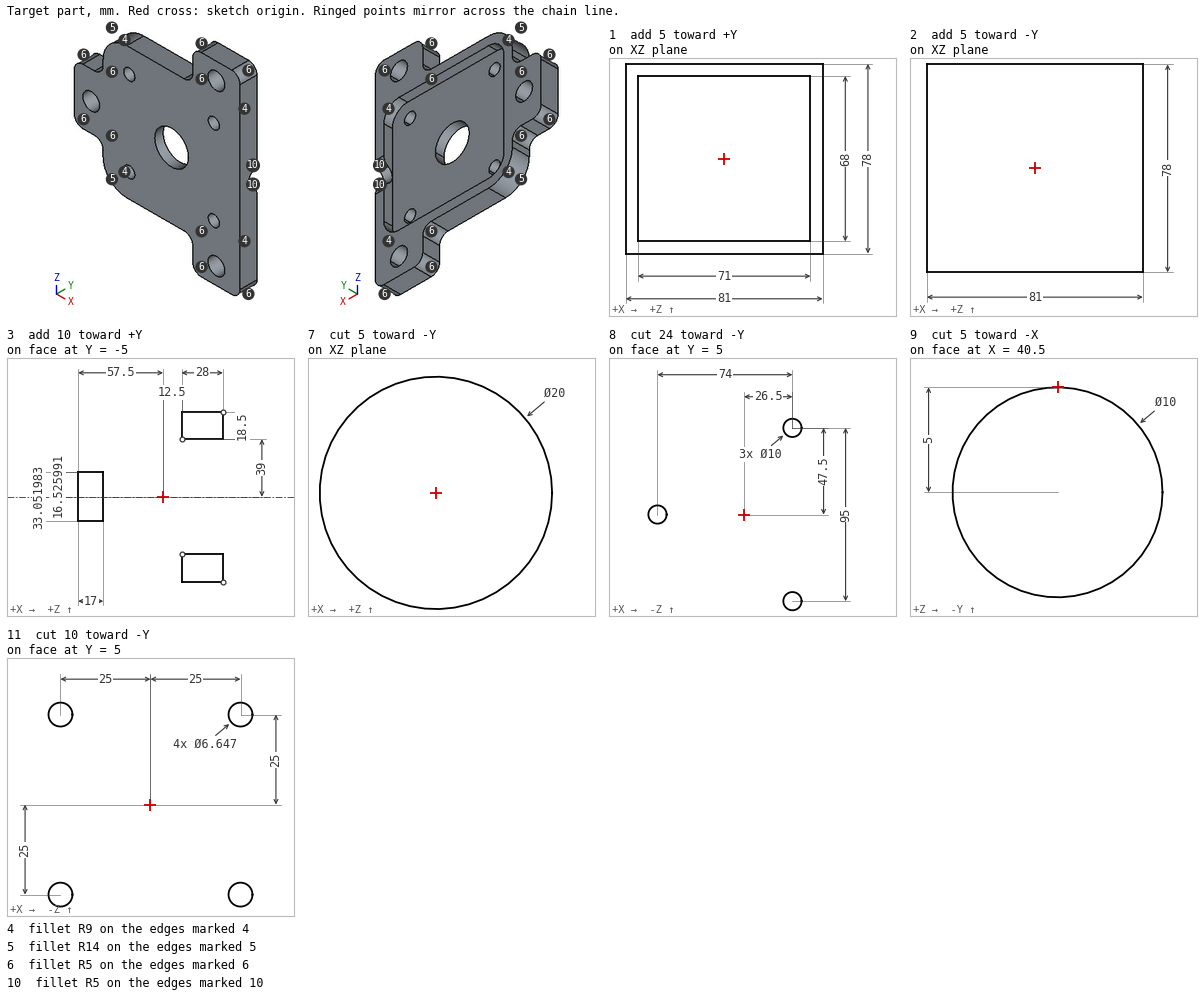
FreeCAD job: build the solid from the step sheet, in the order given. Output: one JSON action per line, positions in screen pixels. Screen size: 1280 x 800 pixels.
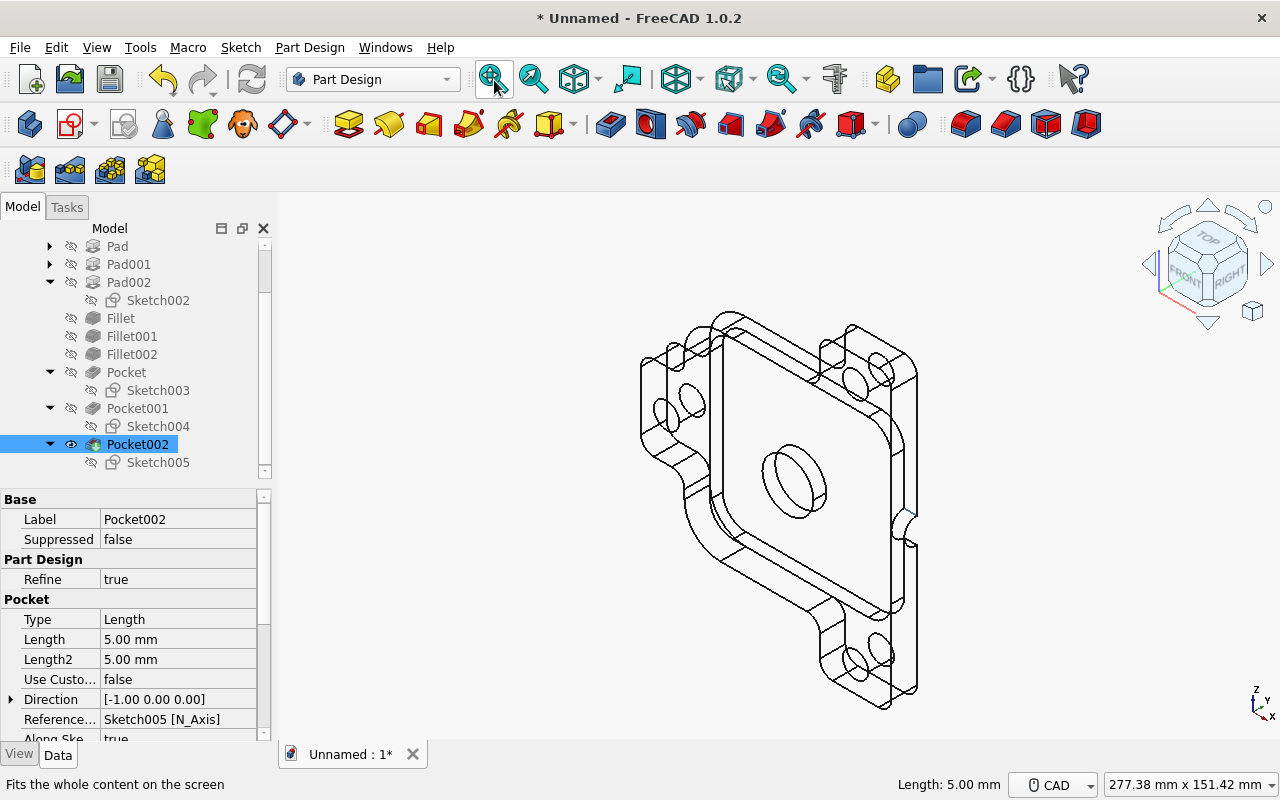
{"action": "scroll", "coordinate": [911, 540], "scroll_direction": "up", "scroll_amount": 4}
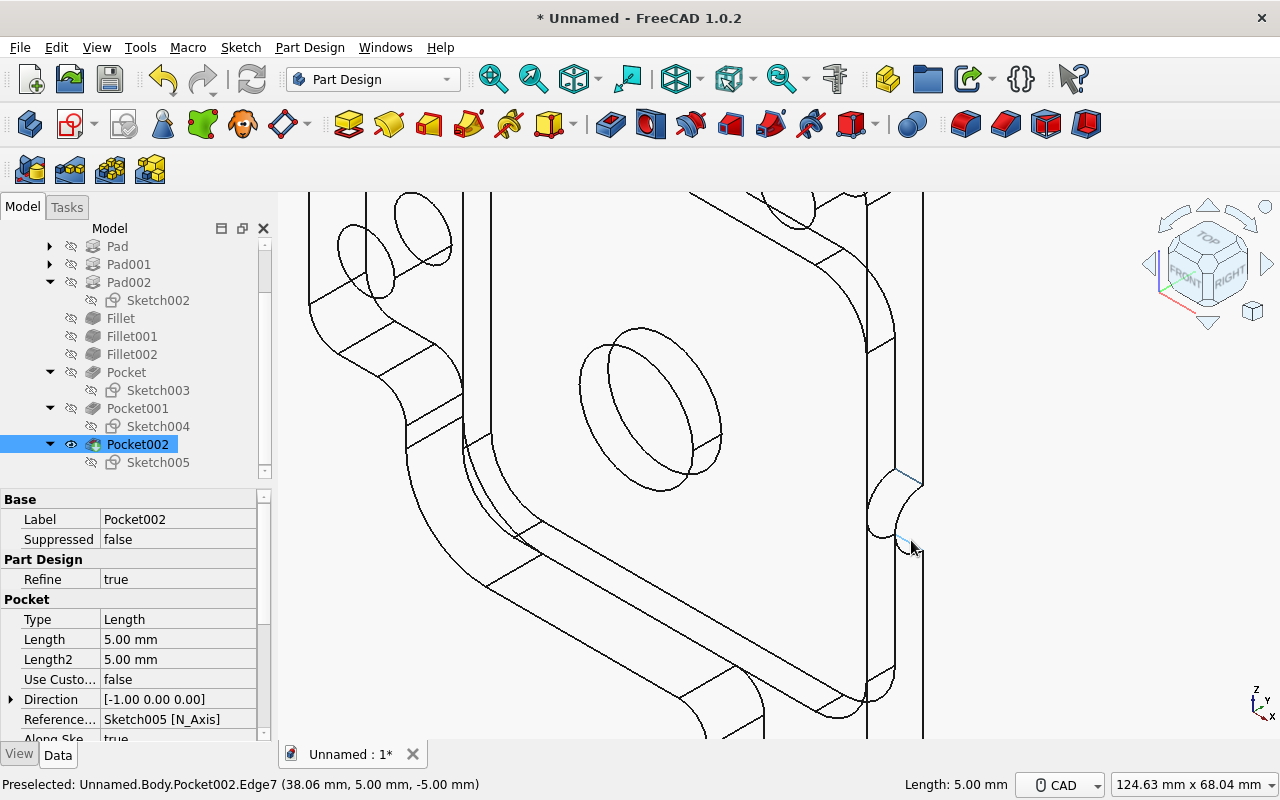
{"action": "left_click", "coordinate": [909, 541], "text": "ctrl"}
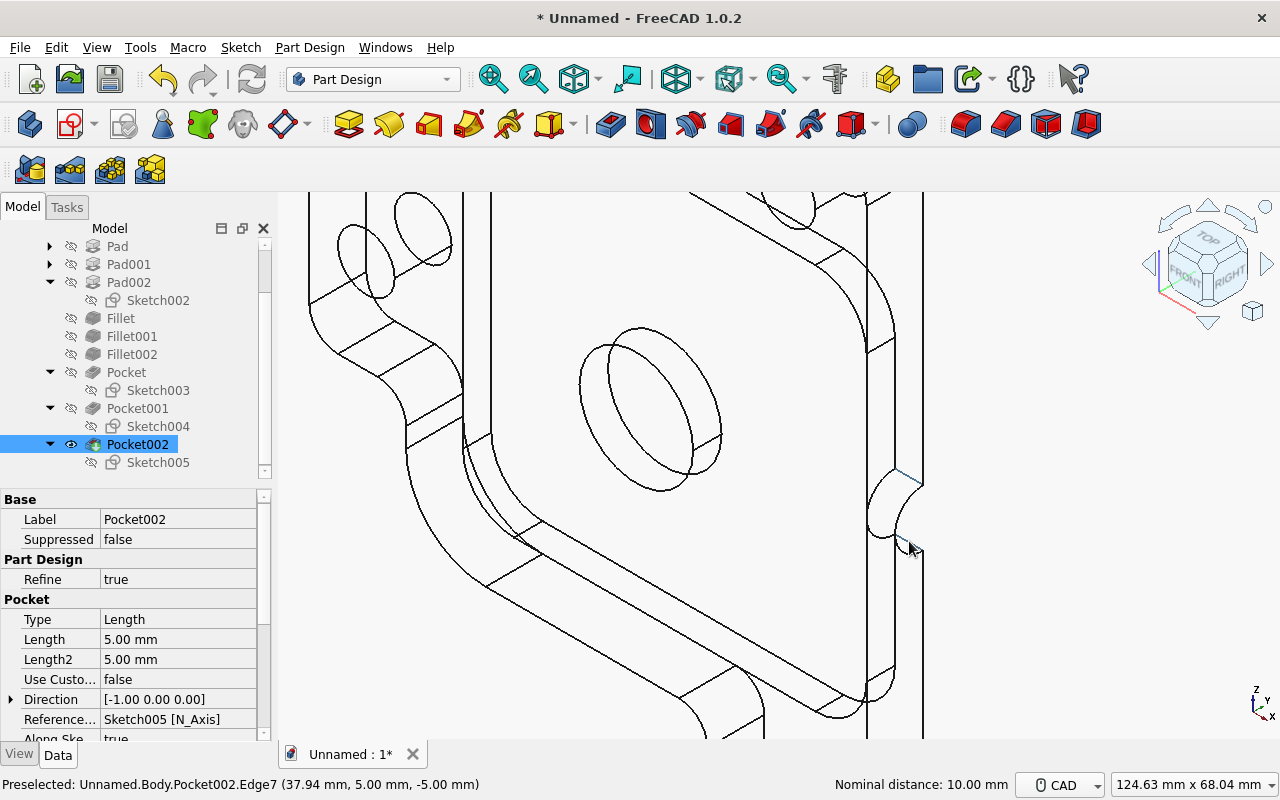
{"action": "key", "text": "v 1"}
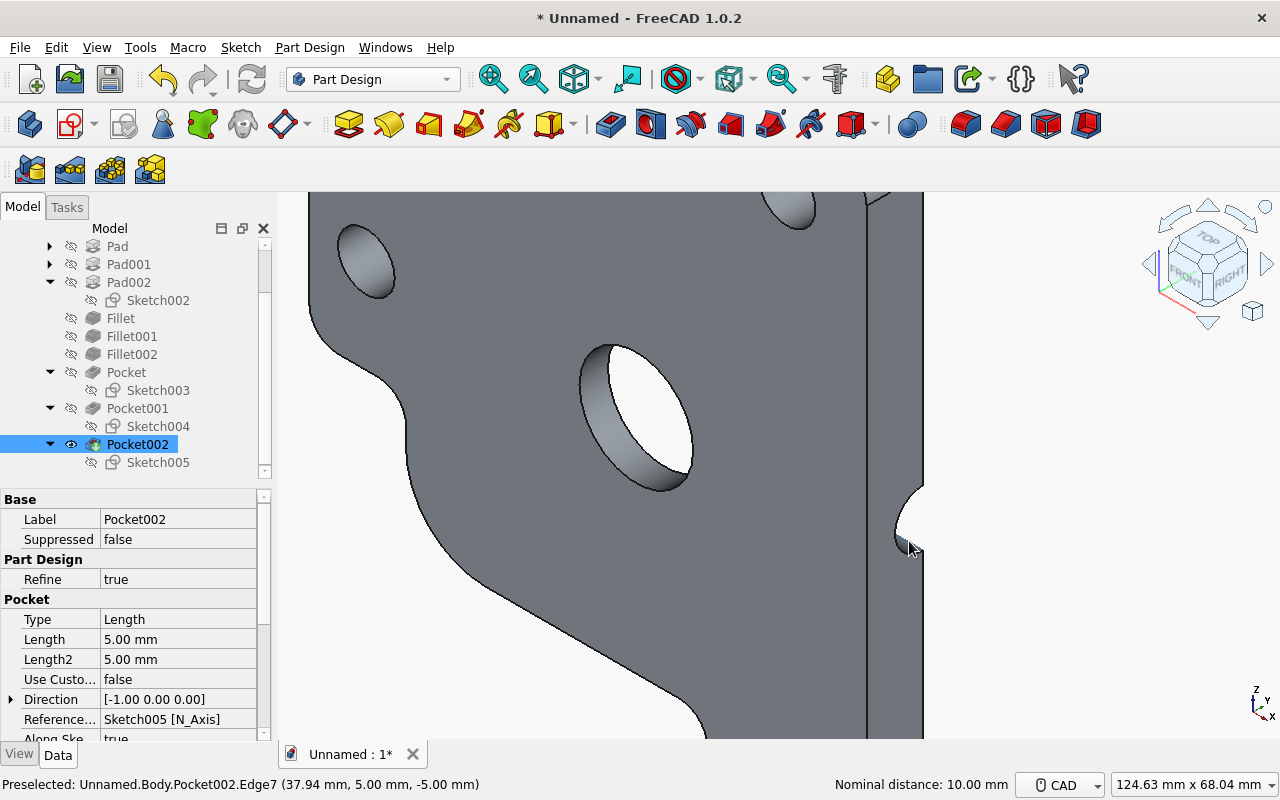
{"action": "left_click", "coordinate": [966, 124]}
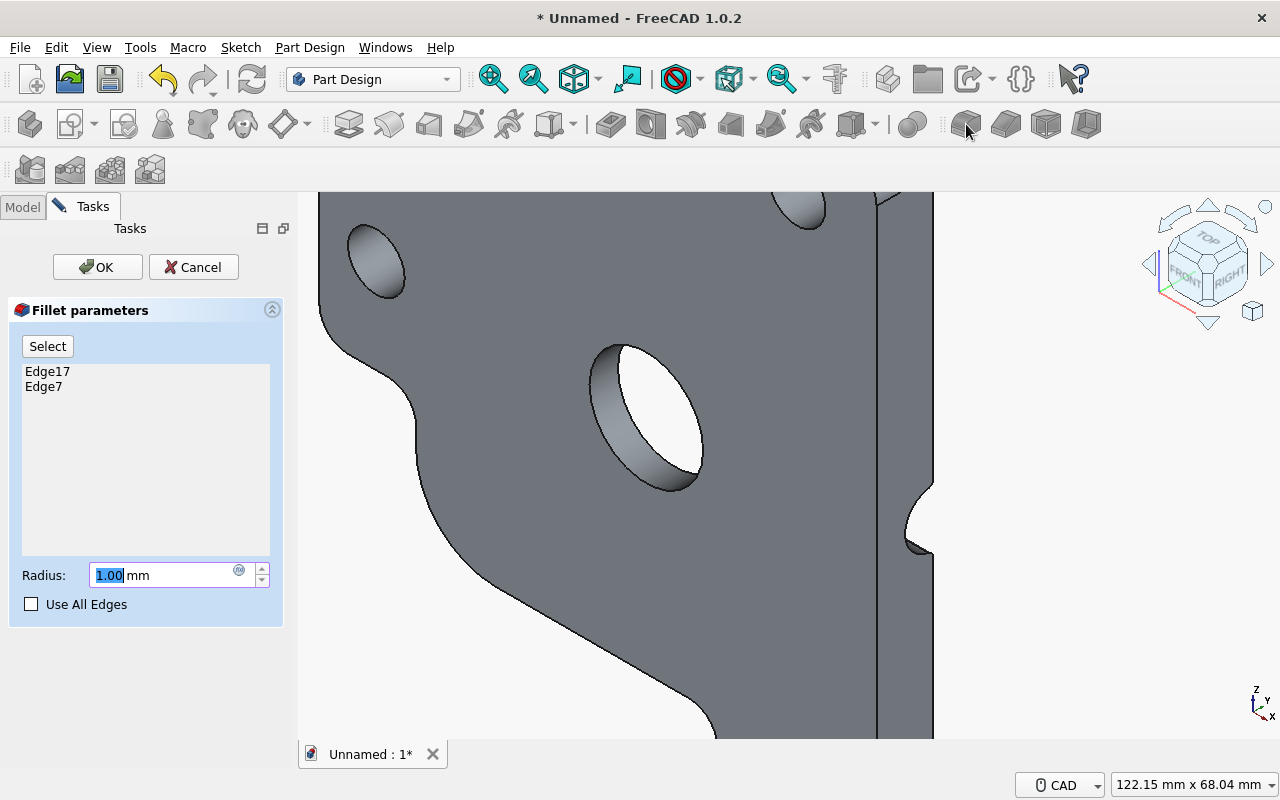
{"action": "type", "text": "5"}
{"action": "key", "text": "Tab"}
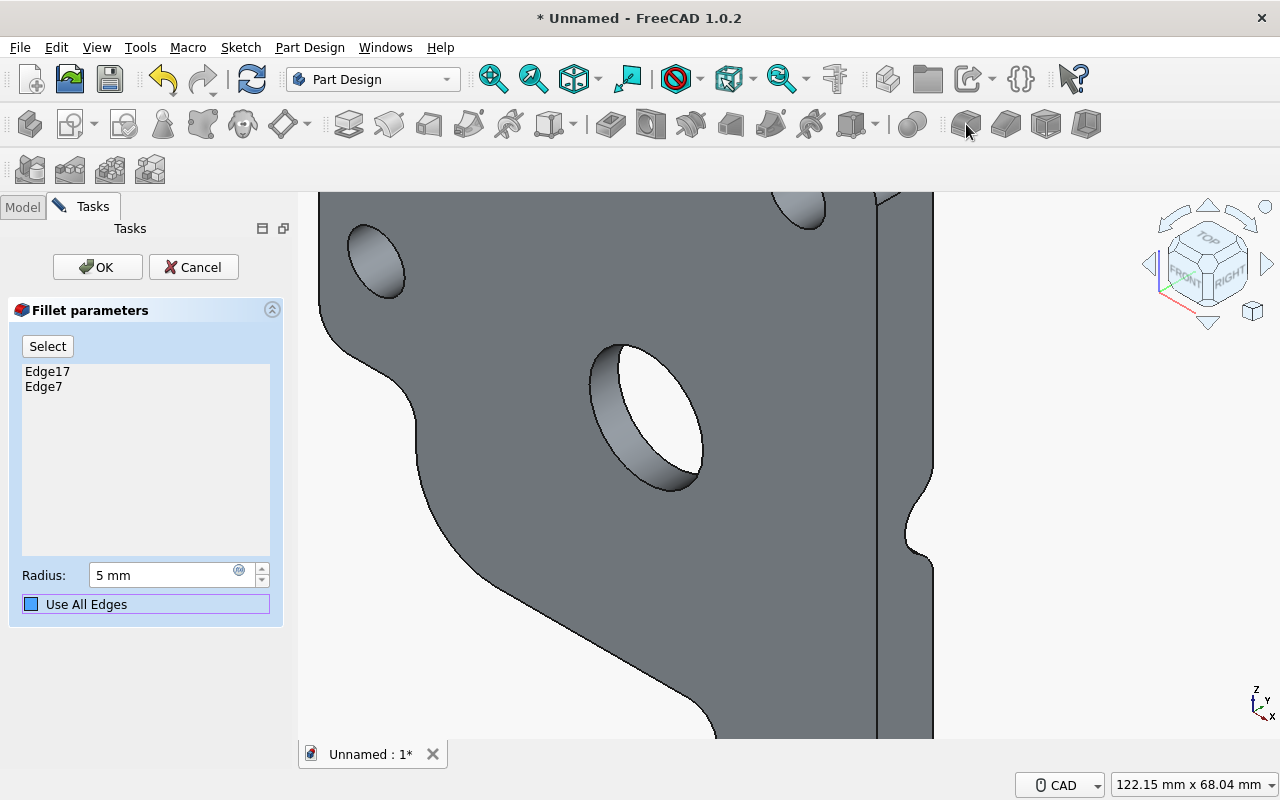
{"action": "left_click", "coordinate": [98, 267]}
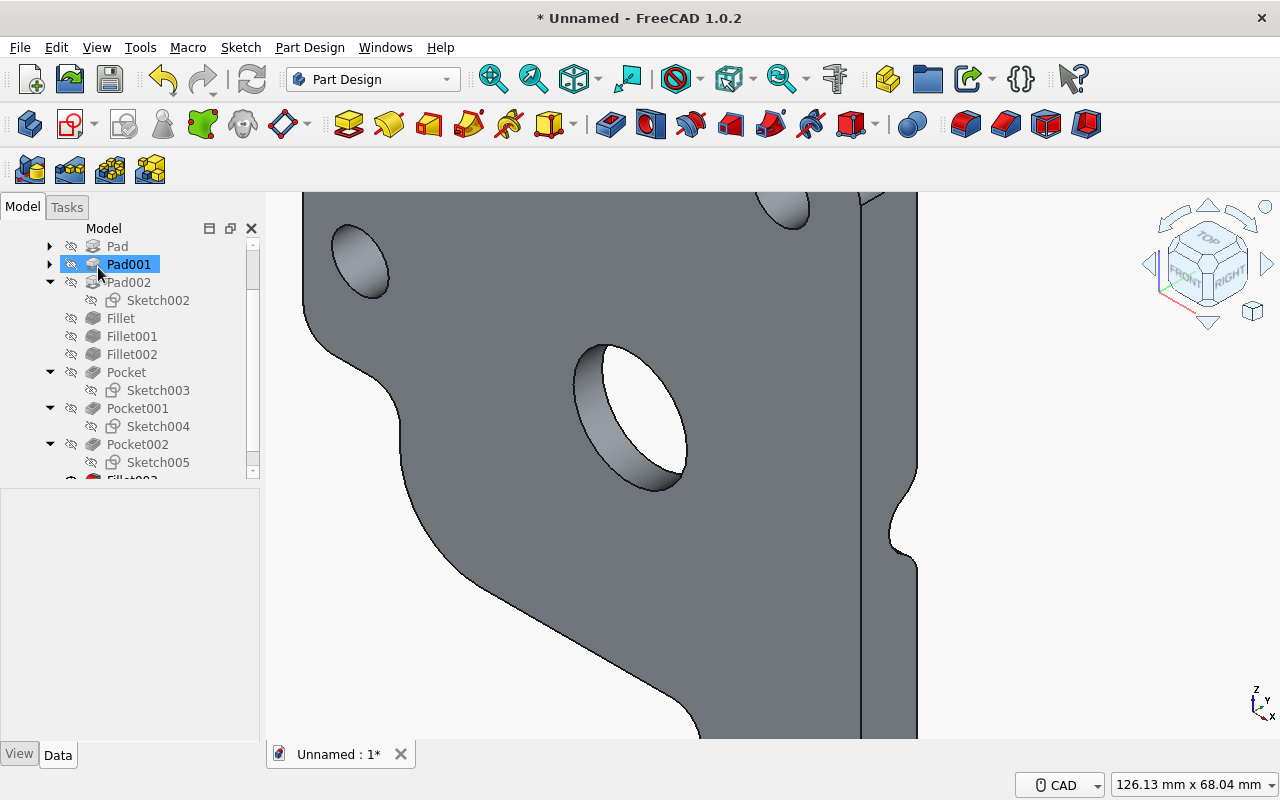
{"action": "key", "text": "v f"}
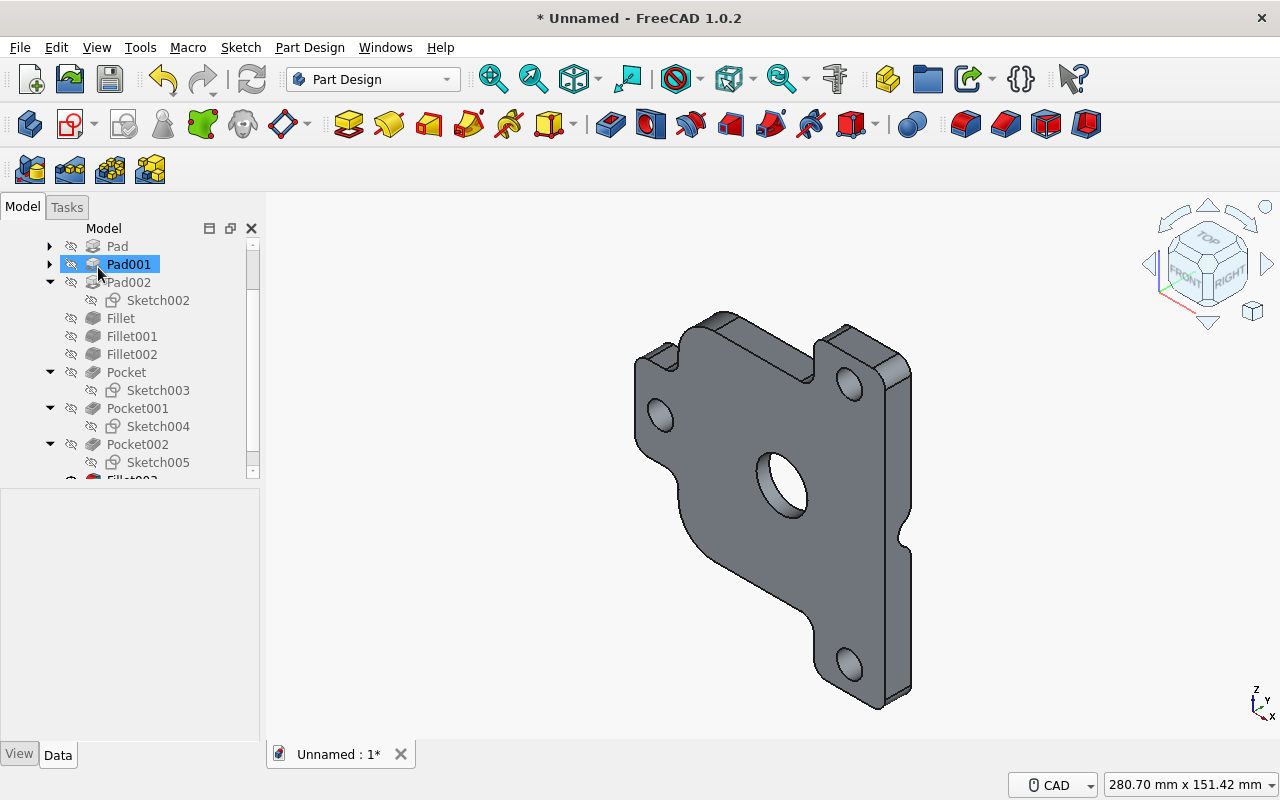
{"action": "key", "text": "4"}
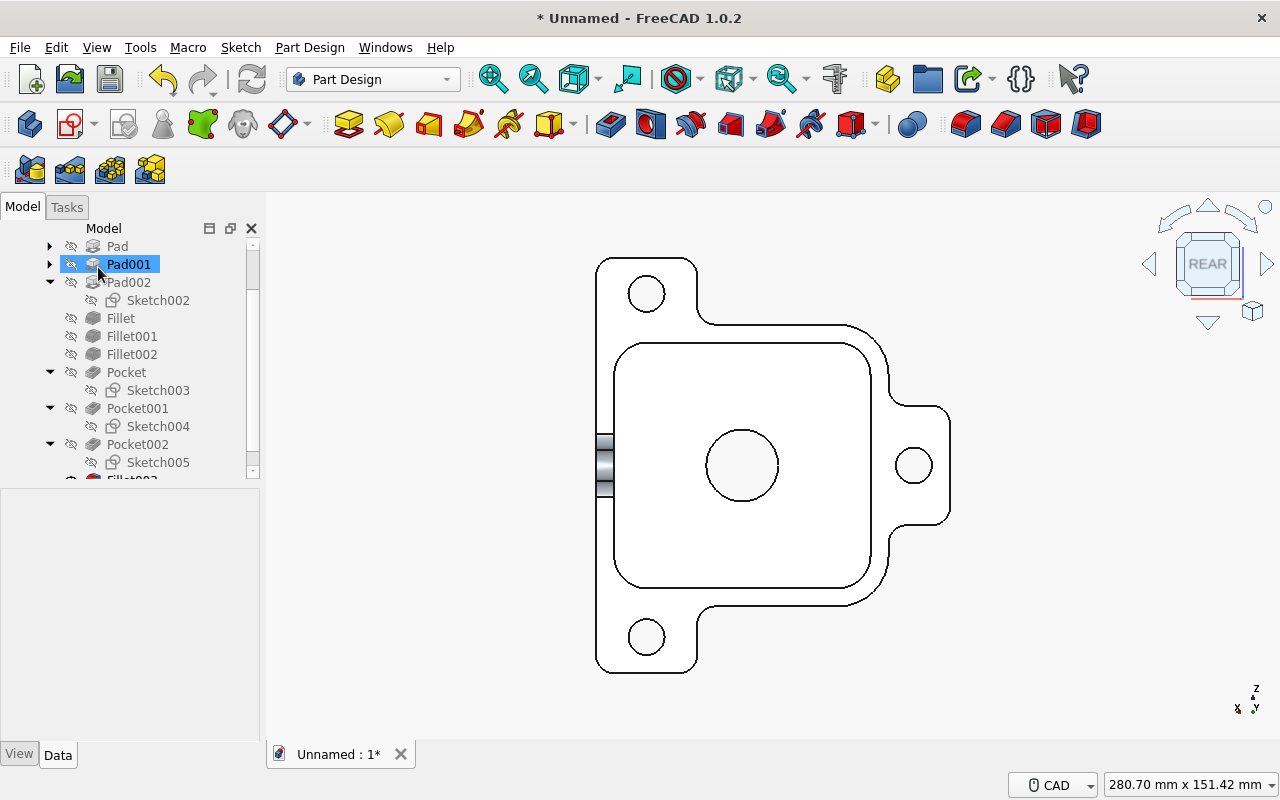
{"action": "left_click", "coordinate": [621, 643]}